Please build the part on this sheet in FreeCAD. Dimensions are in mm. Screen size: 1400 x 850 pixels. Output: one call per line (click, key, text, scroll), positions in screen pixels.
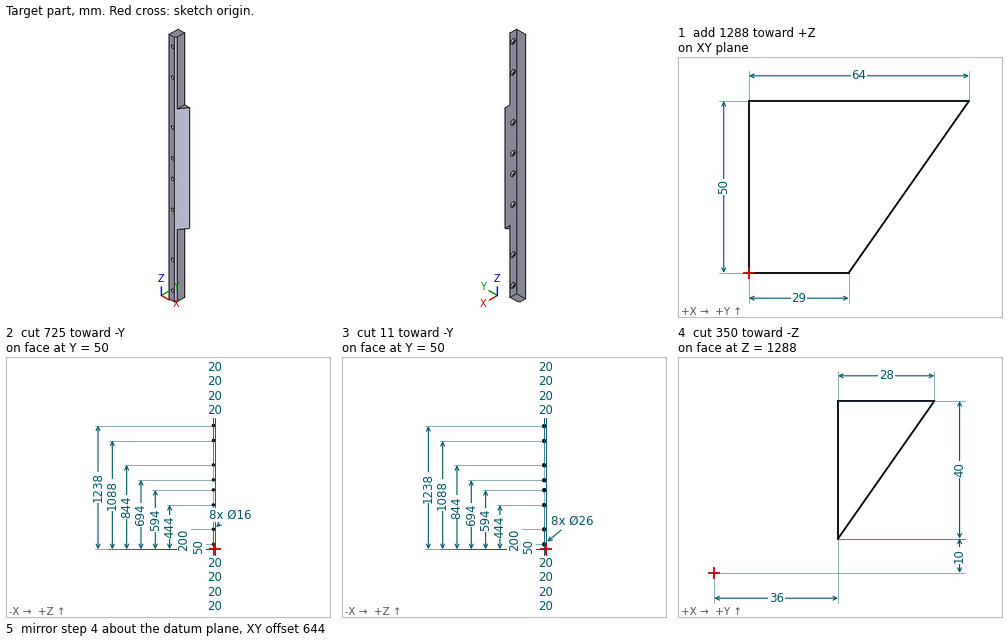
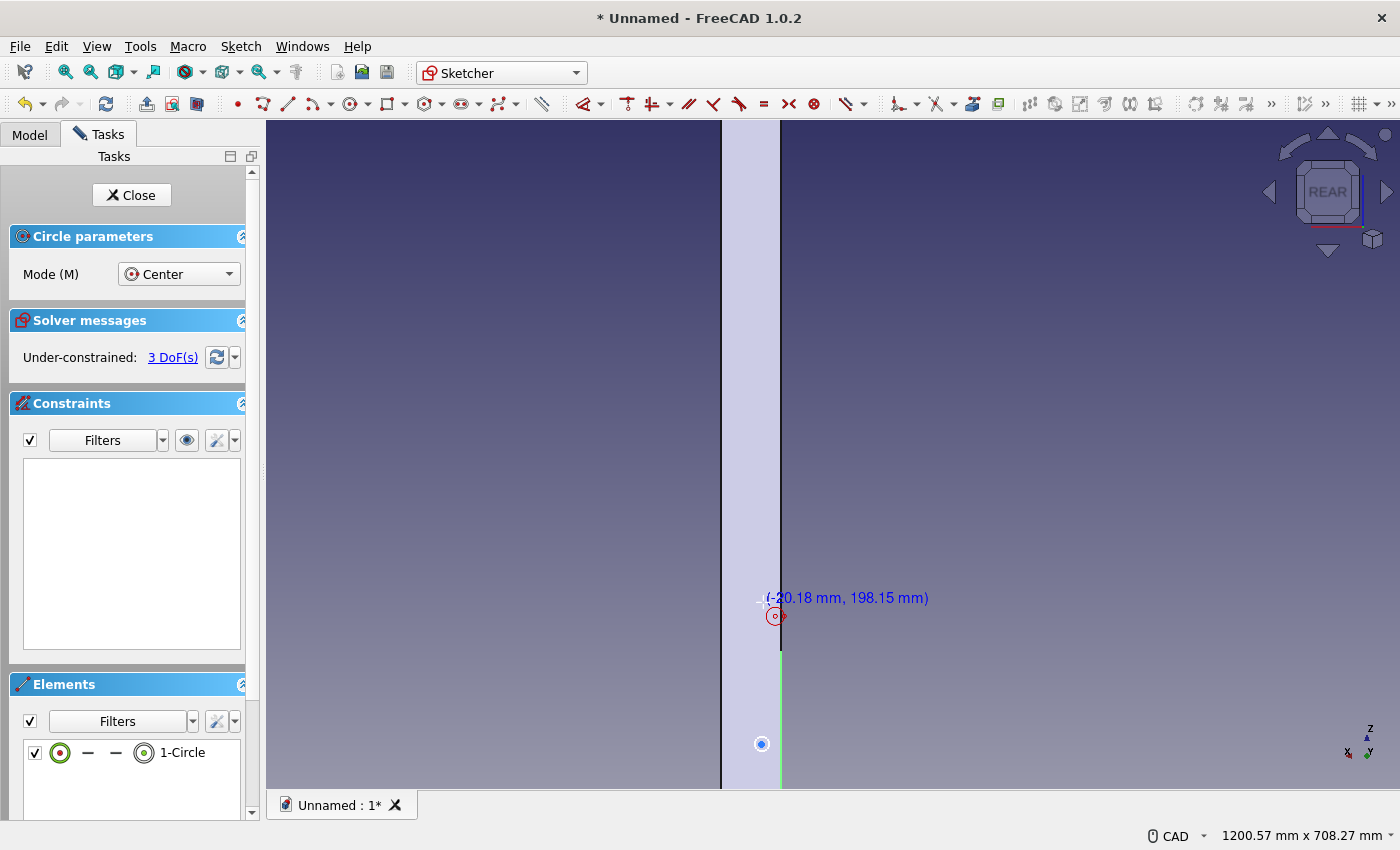
click(762, 602)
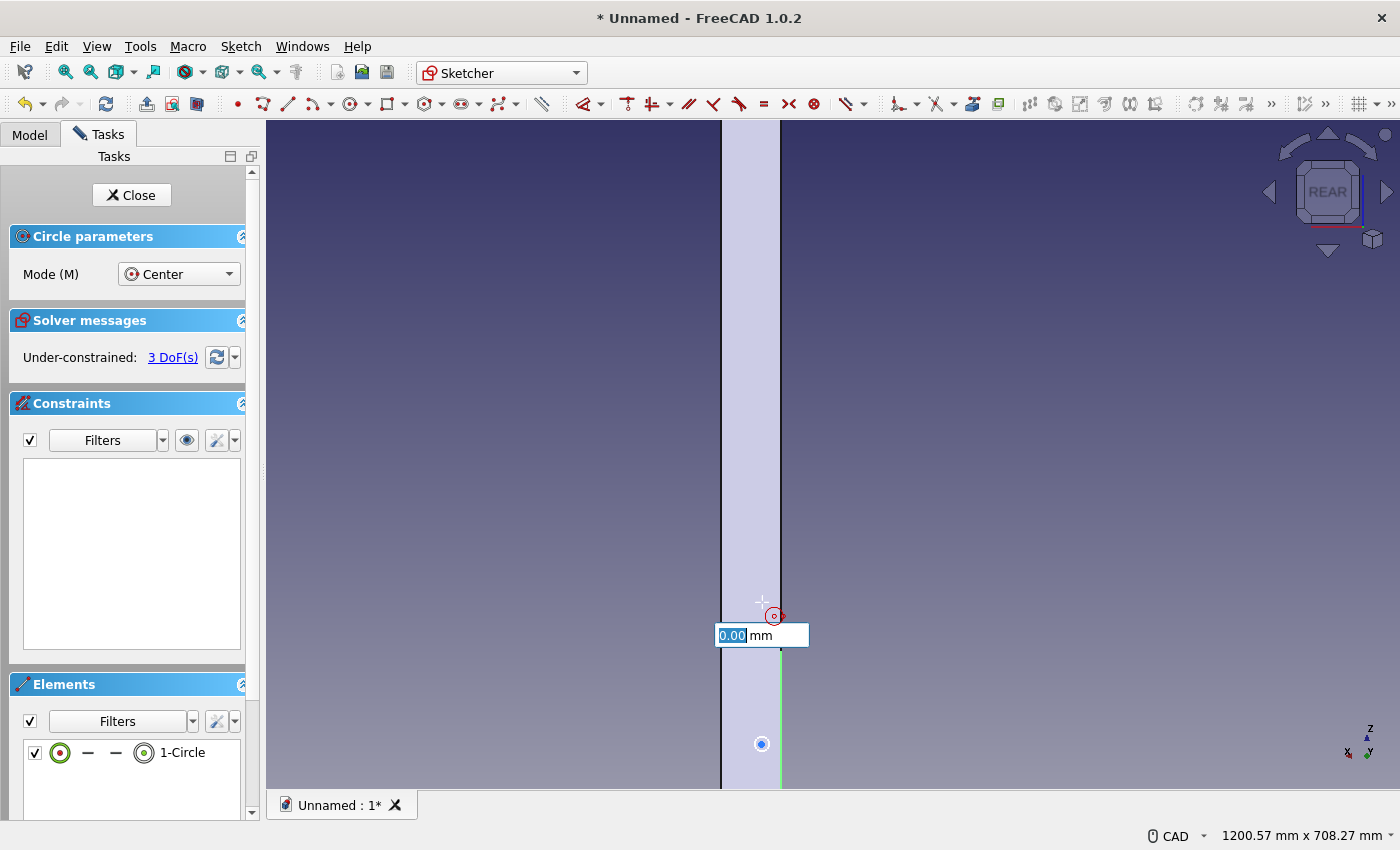
scroll(757, 596, up, 4)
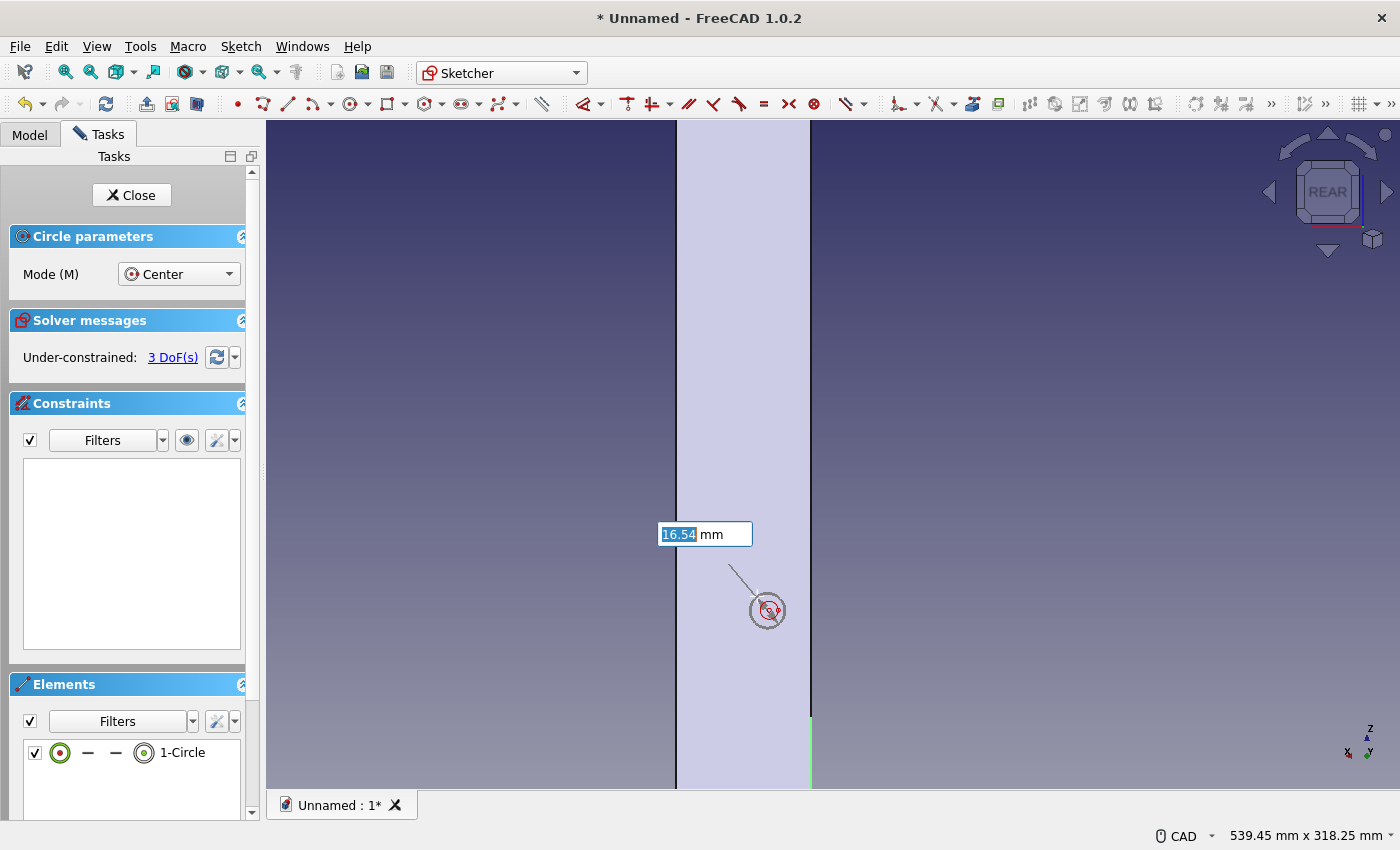
click(757, 596)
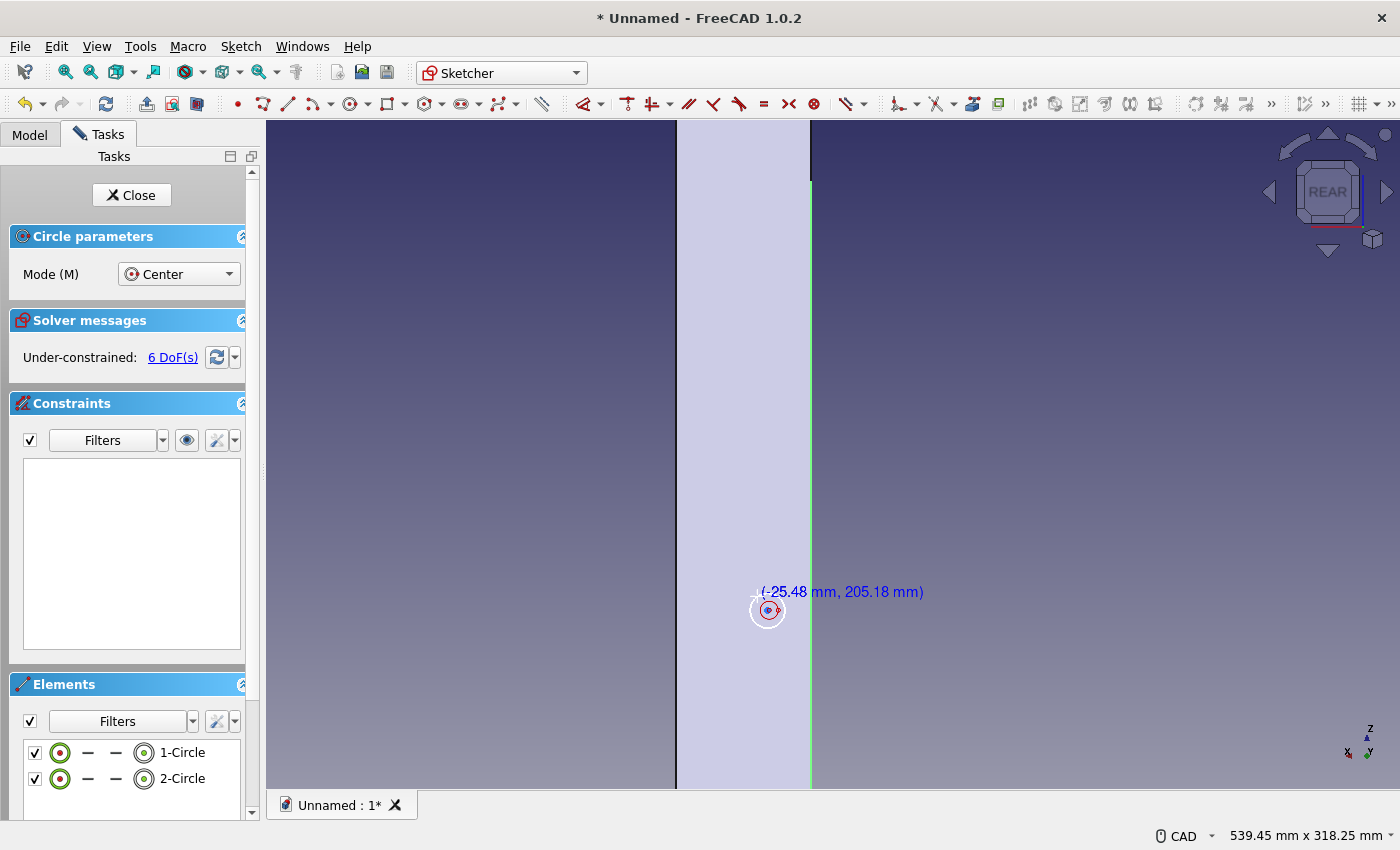
scroll(761, 600, down, 9)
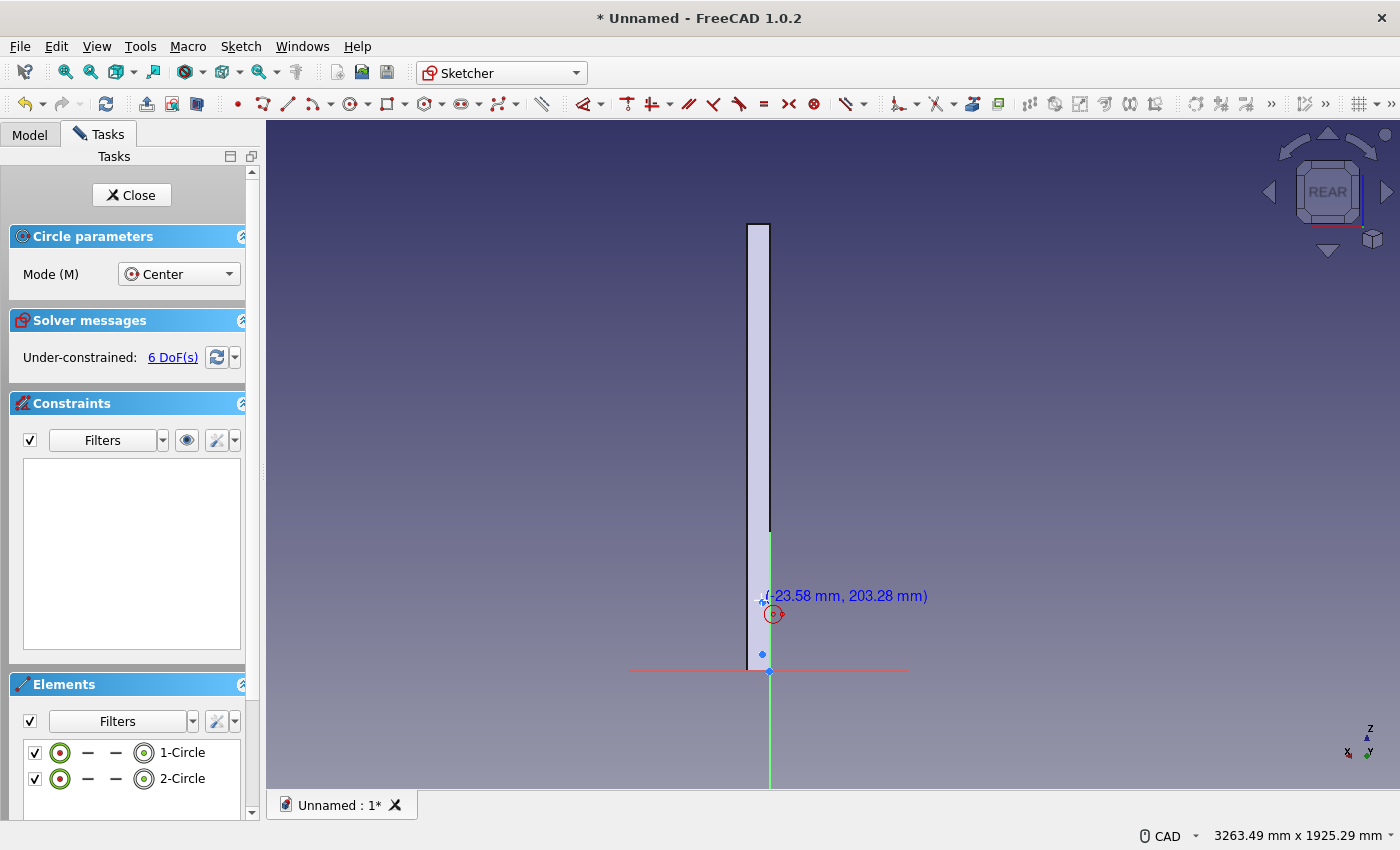
scroll(763, 517, up, 11)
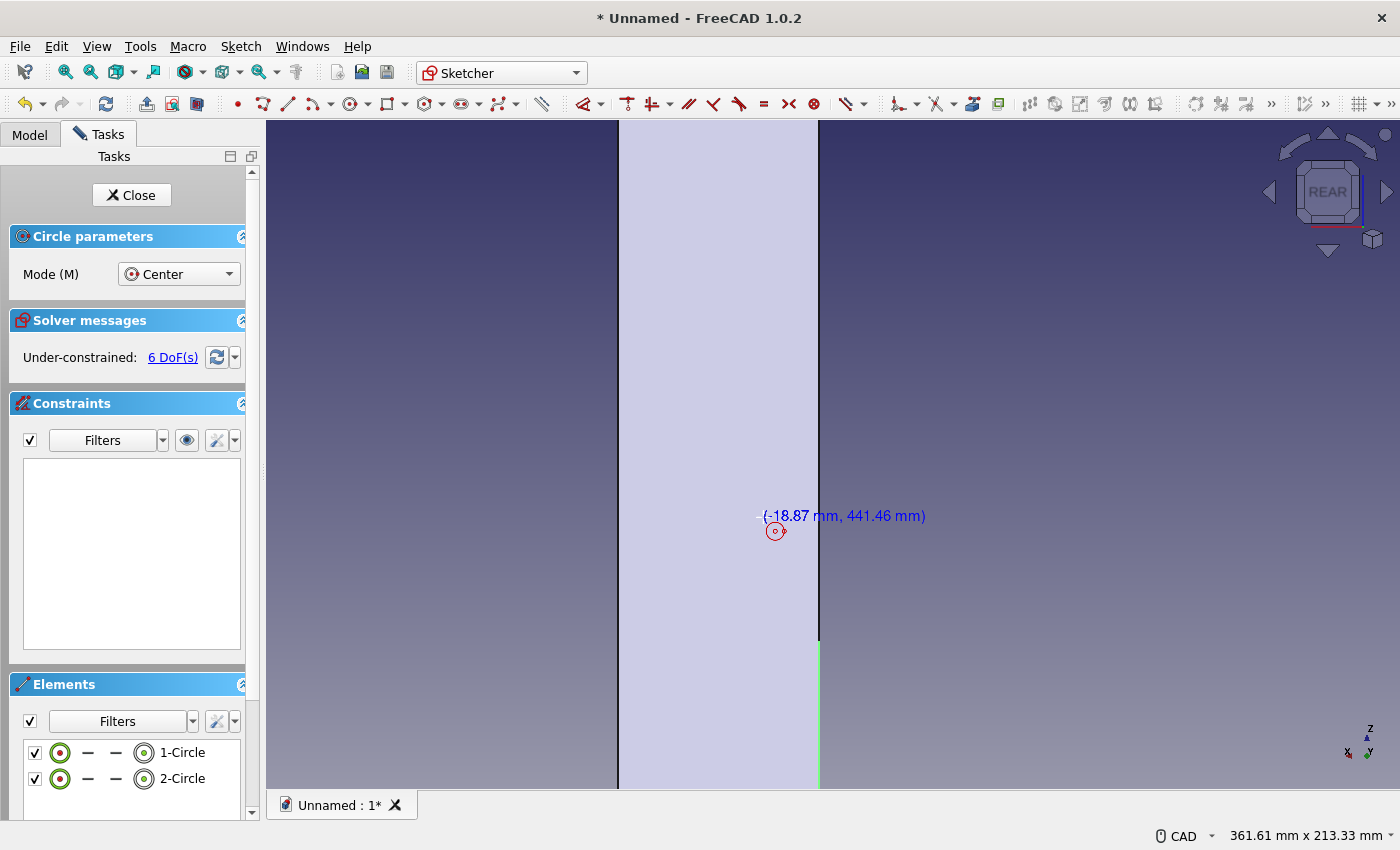
scroll(763, 517, down, 11)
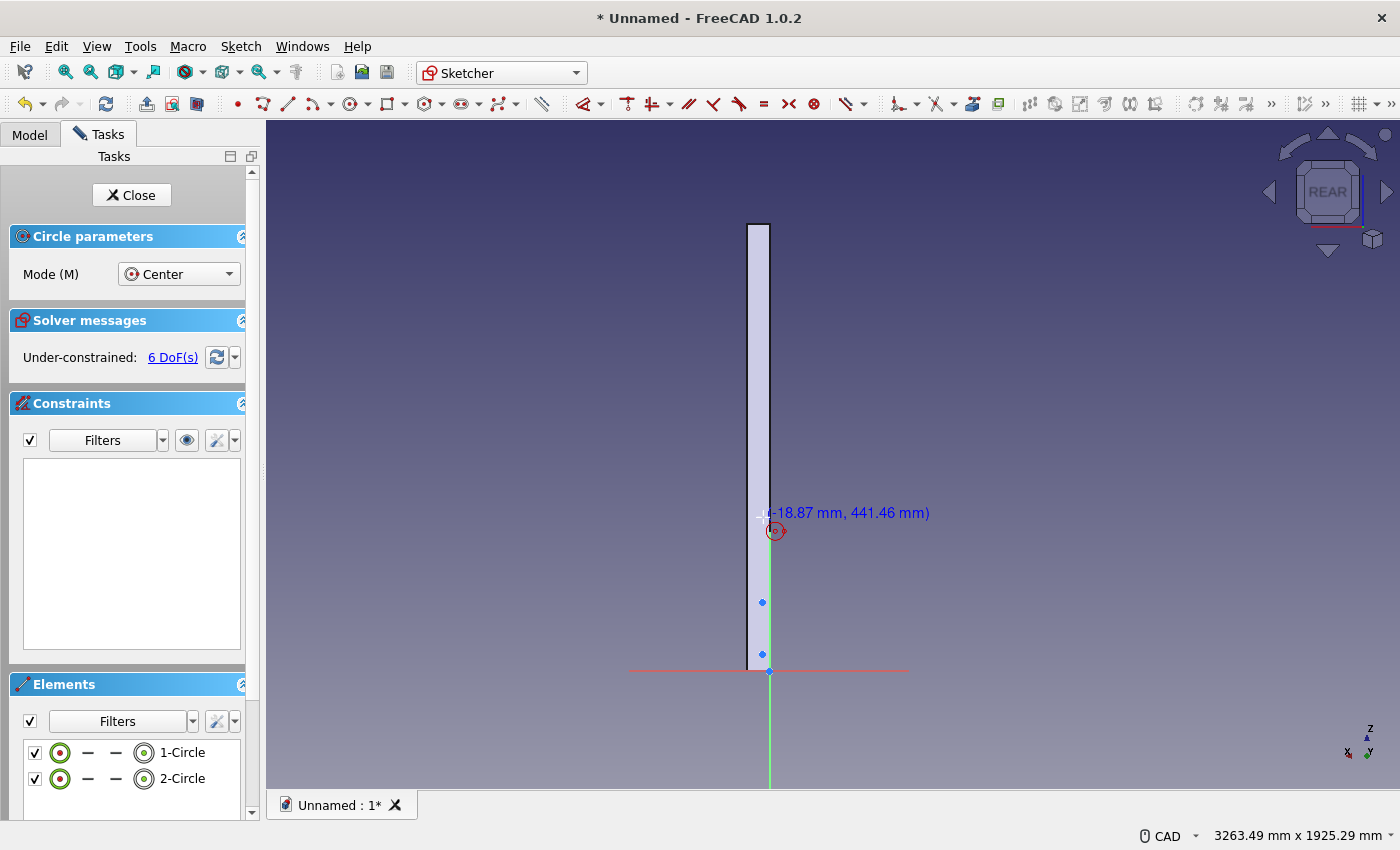
scroll(763, 517, up, 5)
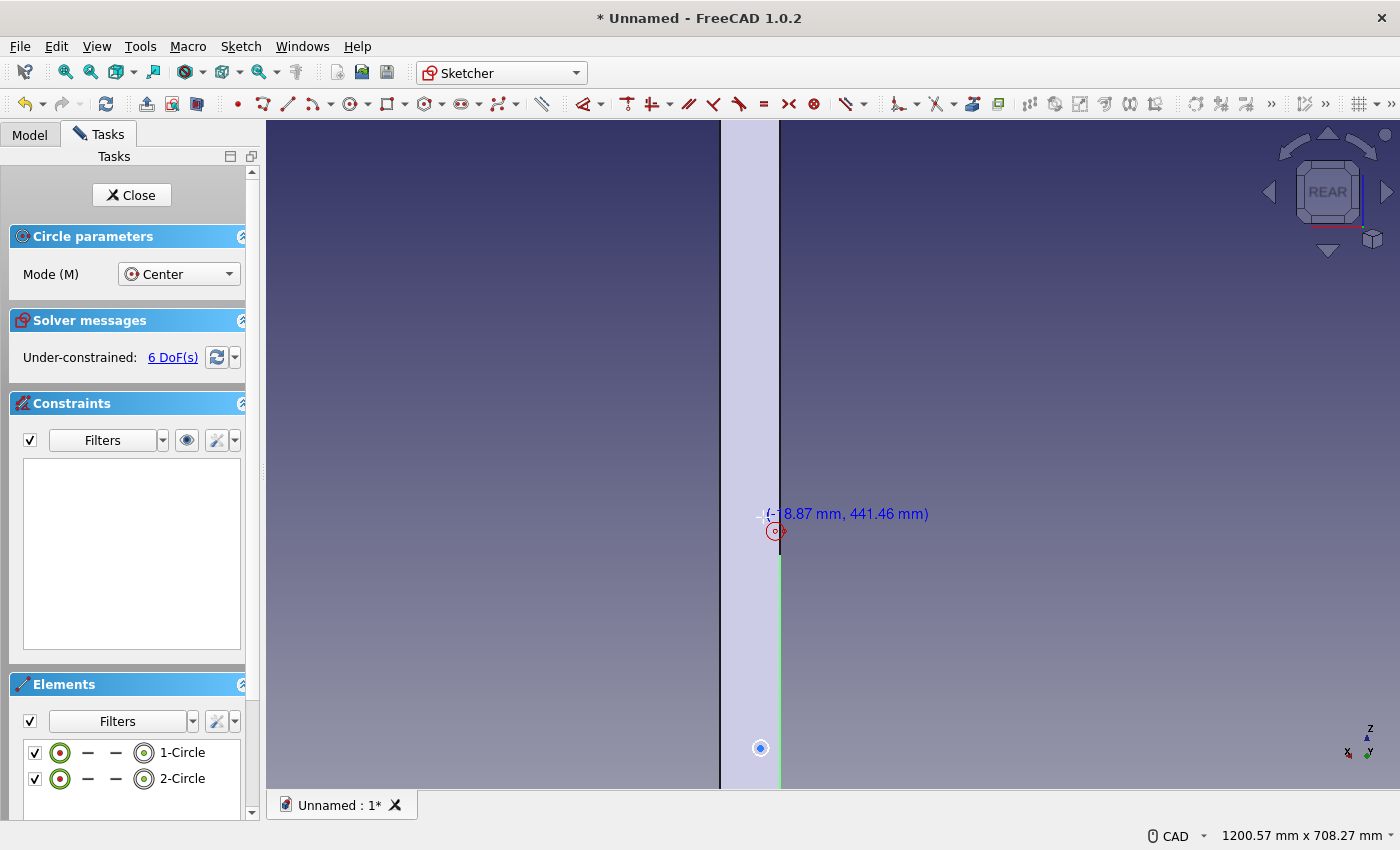
click(761, 516)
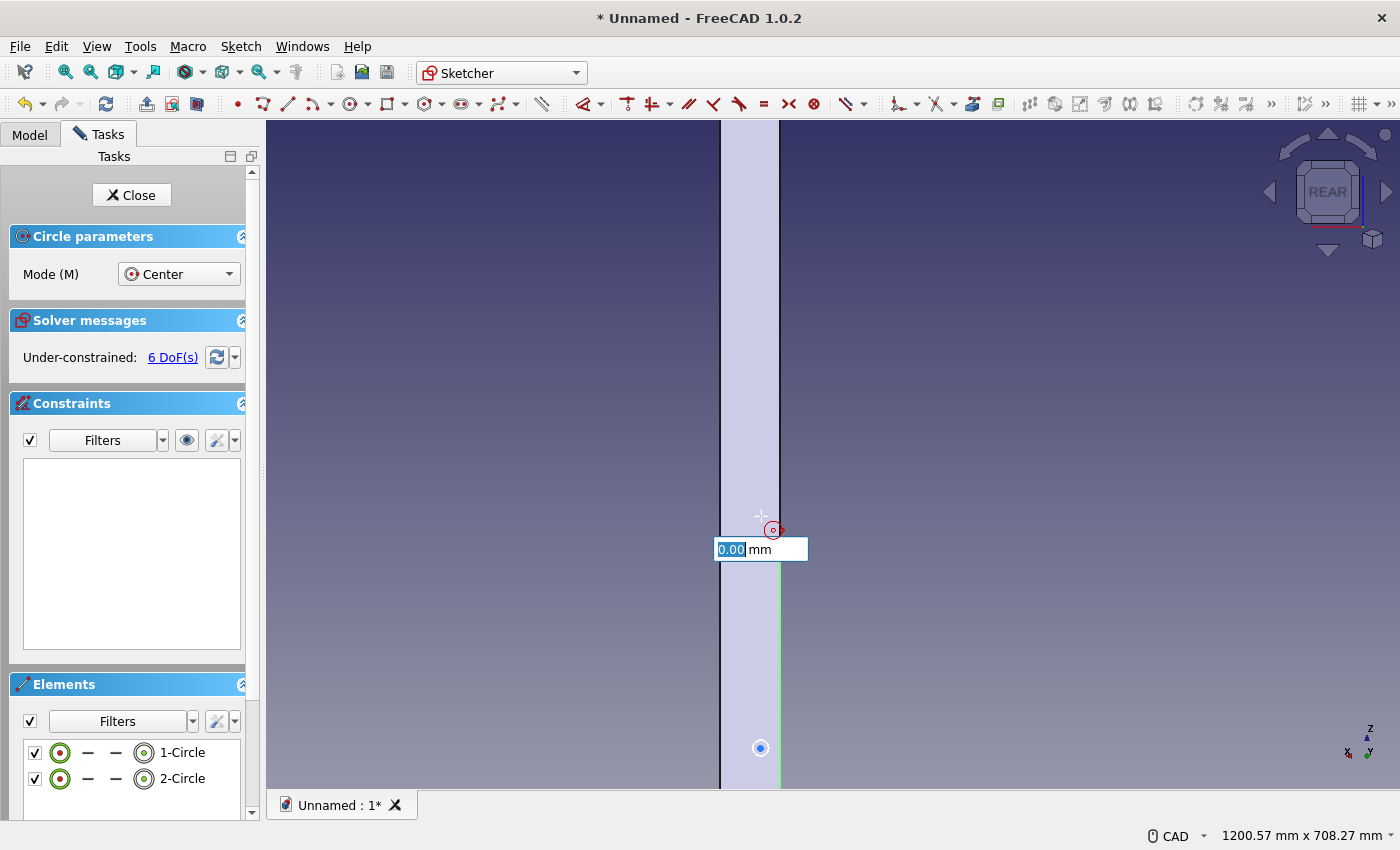
scroll(756, 511, up, 4)